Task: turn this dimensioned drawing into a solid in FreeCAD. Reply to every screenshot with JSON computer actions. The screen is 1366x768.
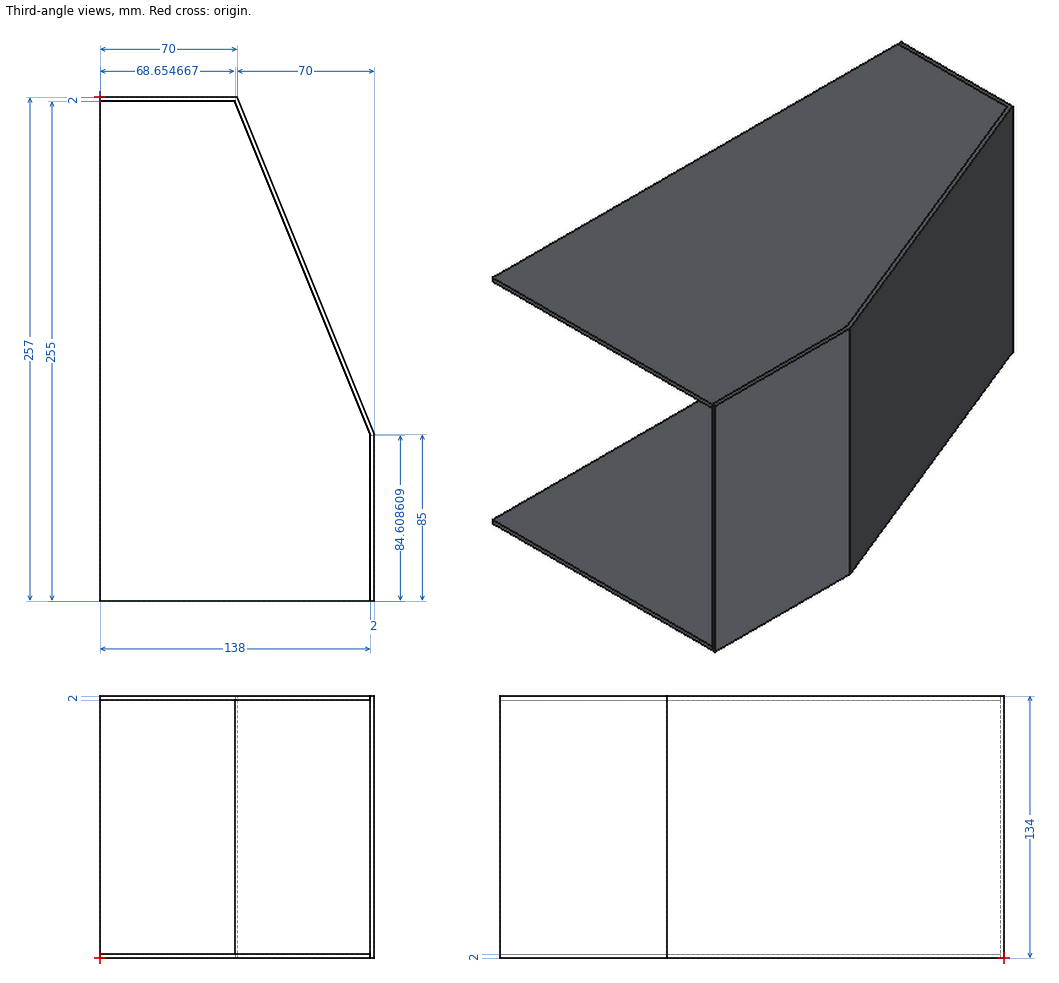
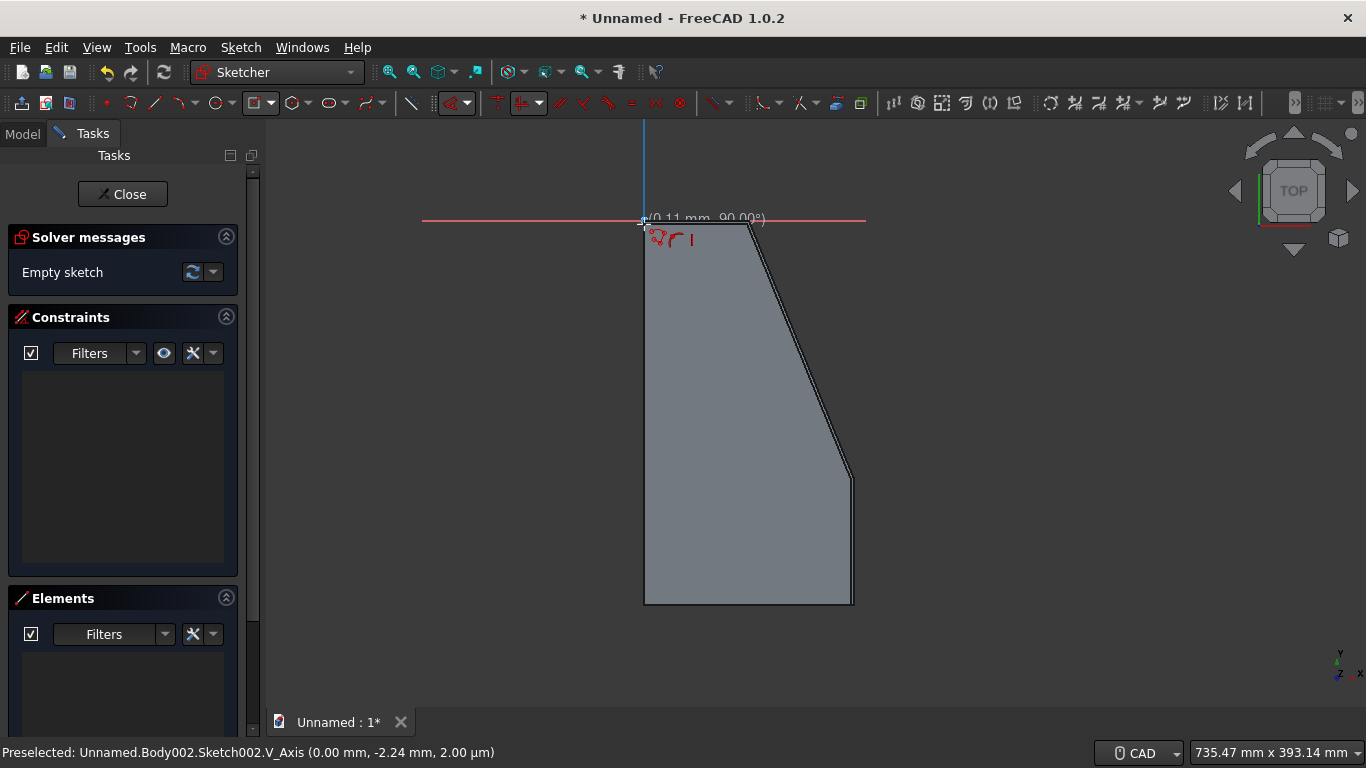
{"action": "left_click", "coordinate": [653, 605]}
{"action": "left_click", "coordinate": [851, 605]}
{"action": "left_click", "coordinate": [851, 479]}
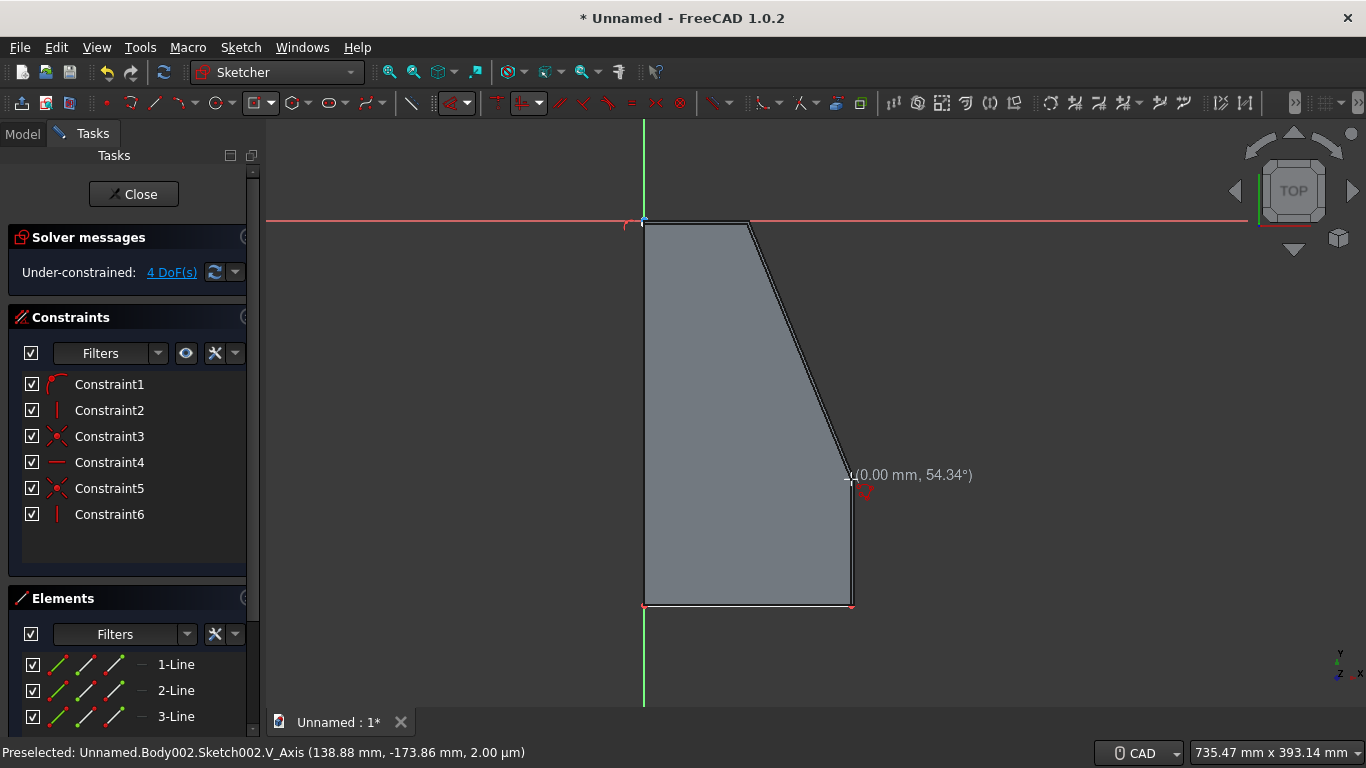
{"action": "scroll", "coordinate": [747, 224], "scroll_direction": "up", "scroll_amount": 9}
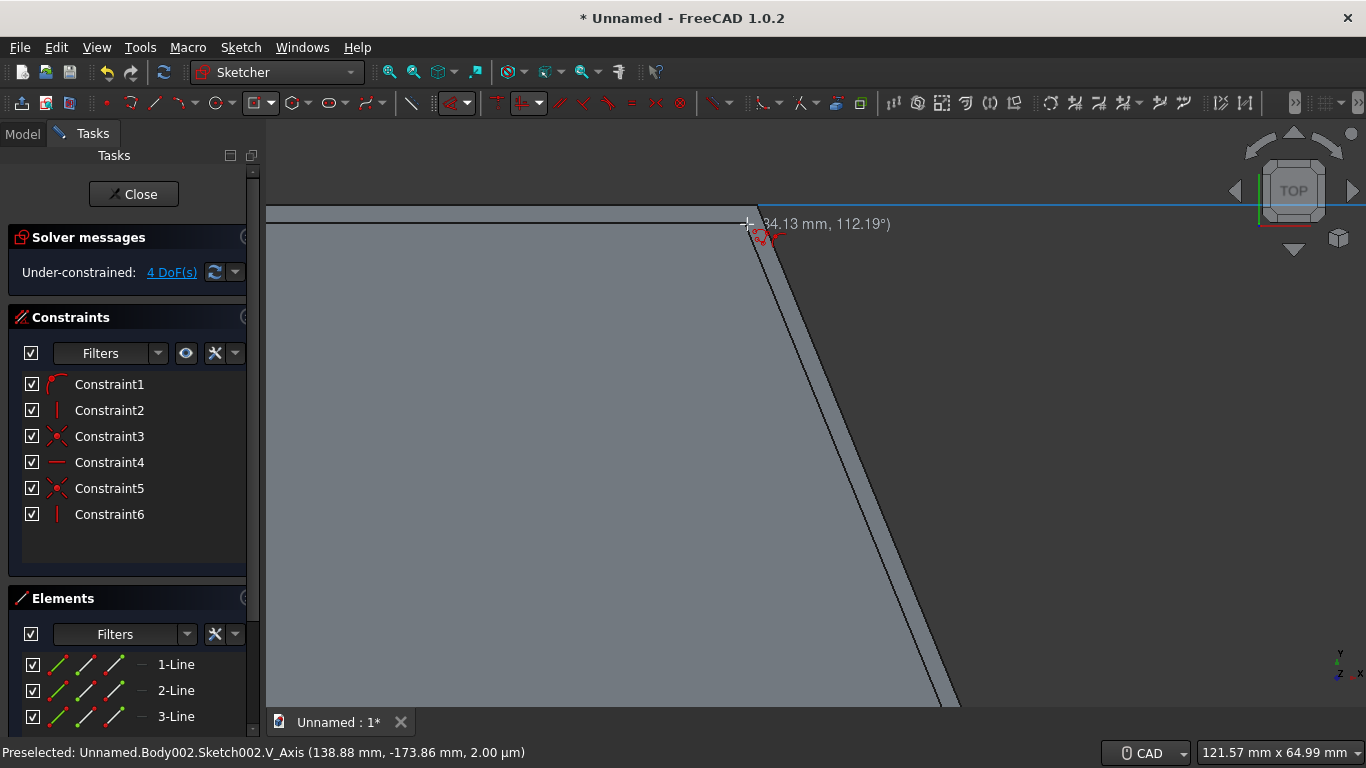
{"action": "left_click", "coordinate": [745, 223]}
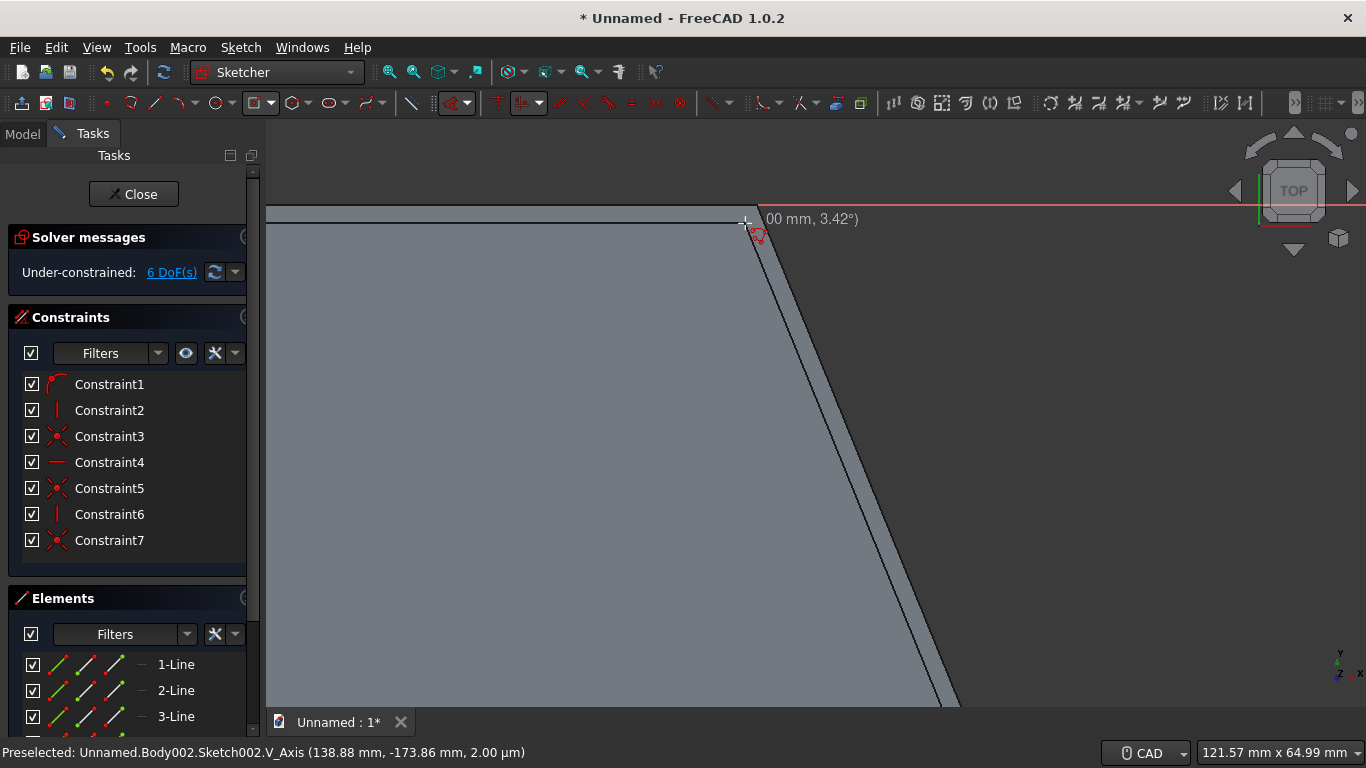
{"action": "scroll", "coordinate": [747, 224], "scroll_direction": "down", "scroll_amount": 9}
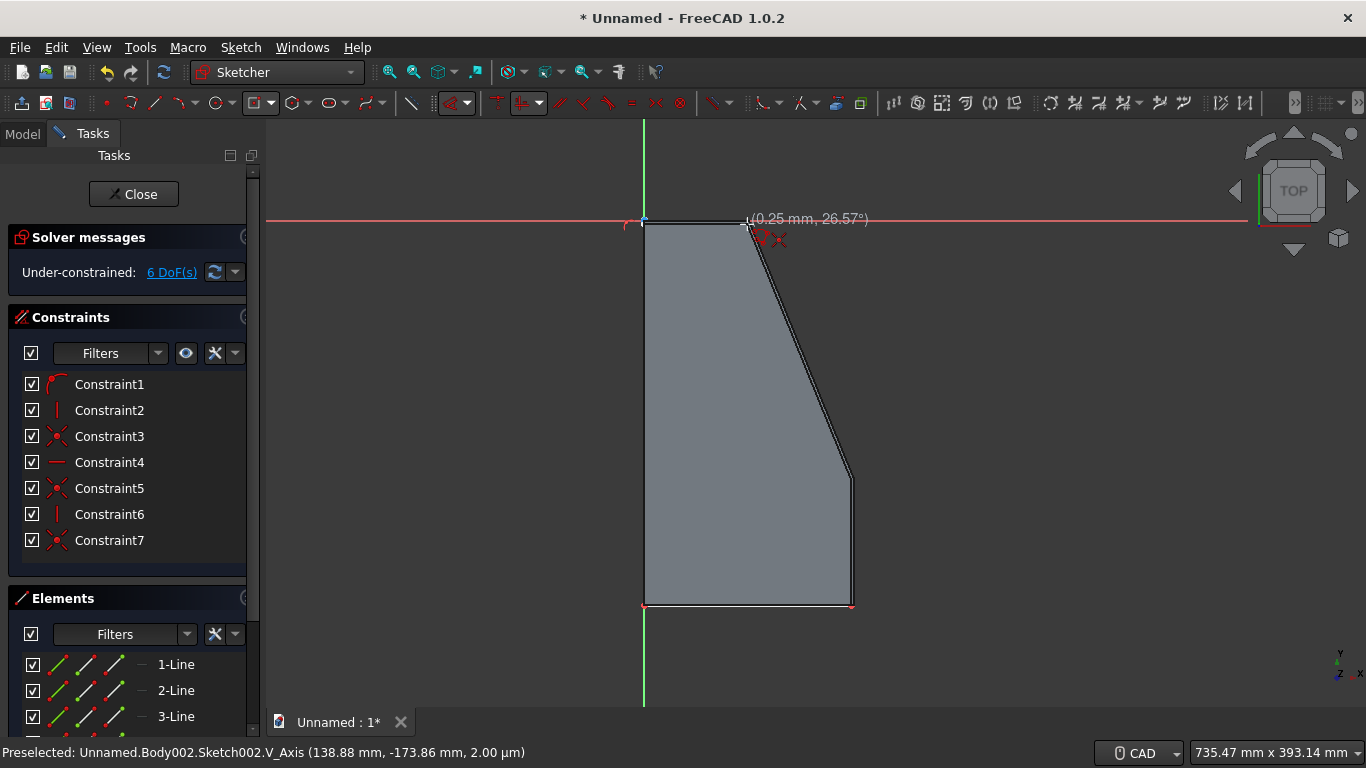
{"action": "scroll", "coordinate": [644, 224], "scroll_direction": "up", "scroll_amount": 9}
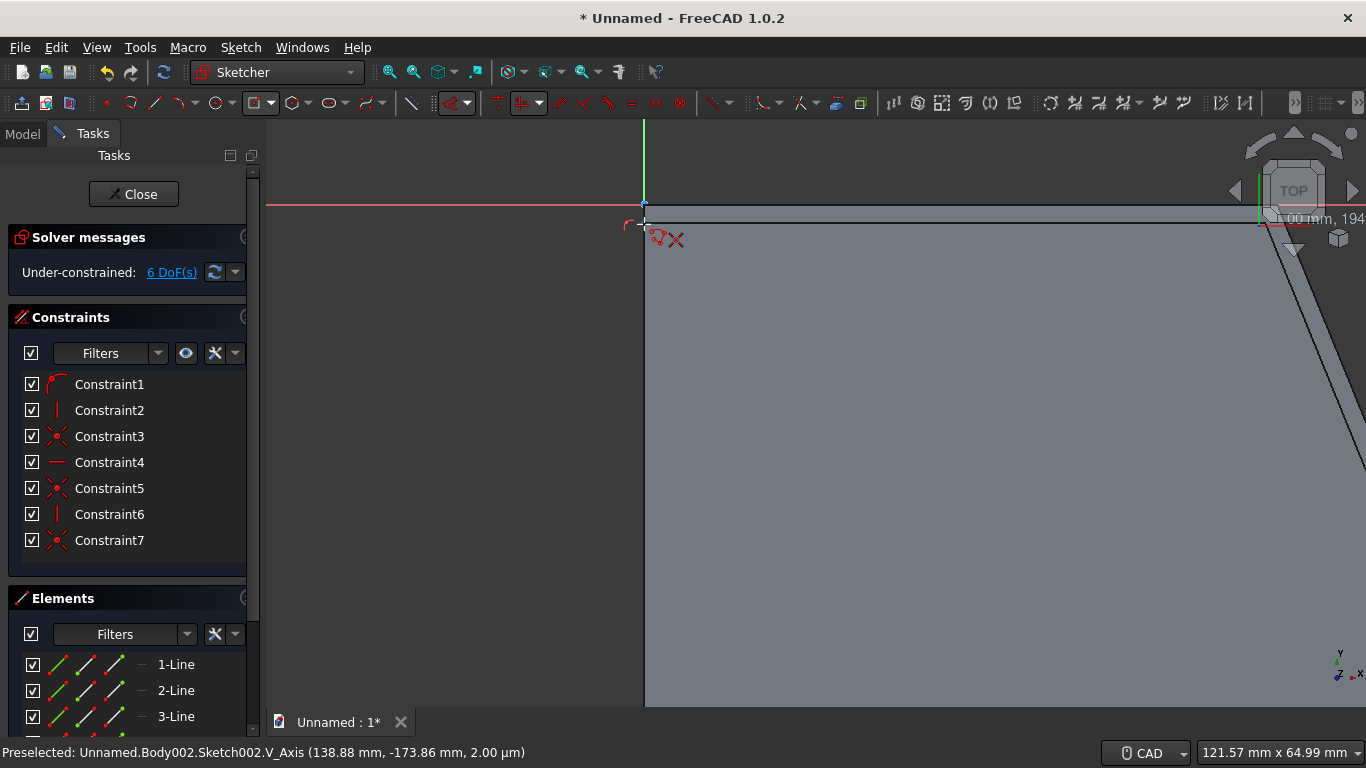
{"action": "left_click", "coordinate": [644, 224]}
{"action": "key", "text": "Escape"}
{"action": "key", "text": "Escape"}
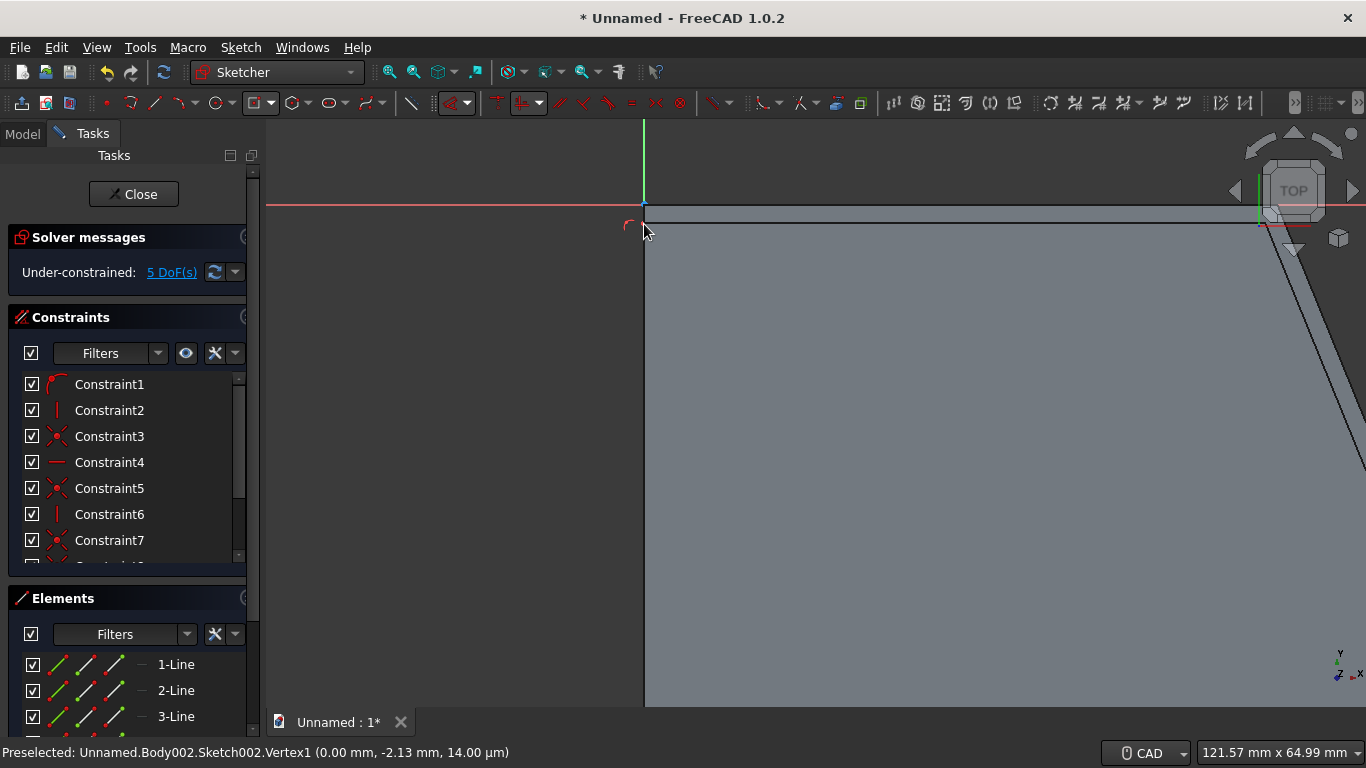
{"action": "key", "text": "d"}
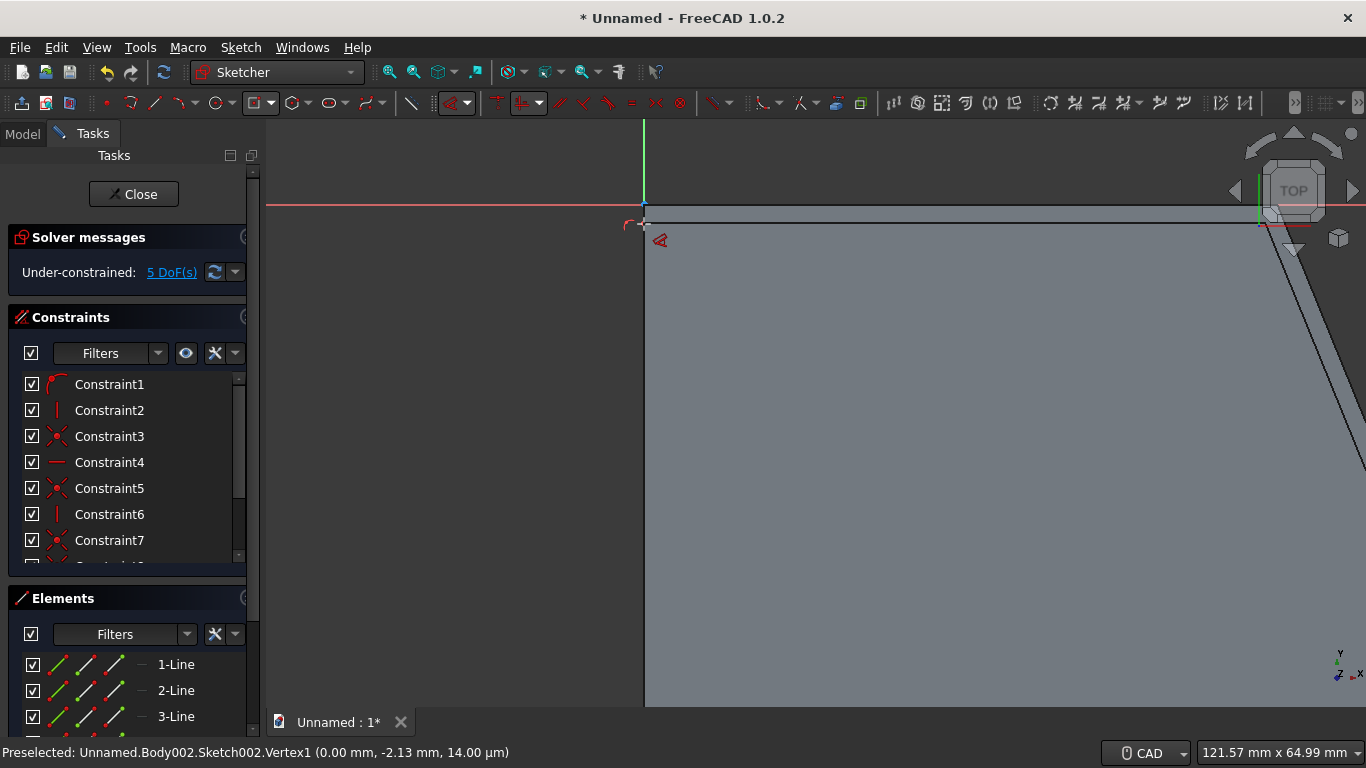
{"action": "scroll", "coordinate": [644, 224], "scroll_direction": "up", "scroll_amount": 4}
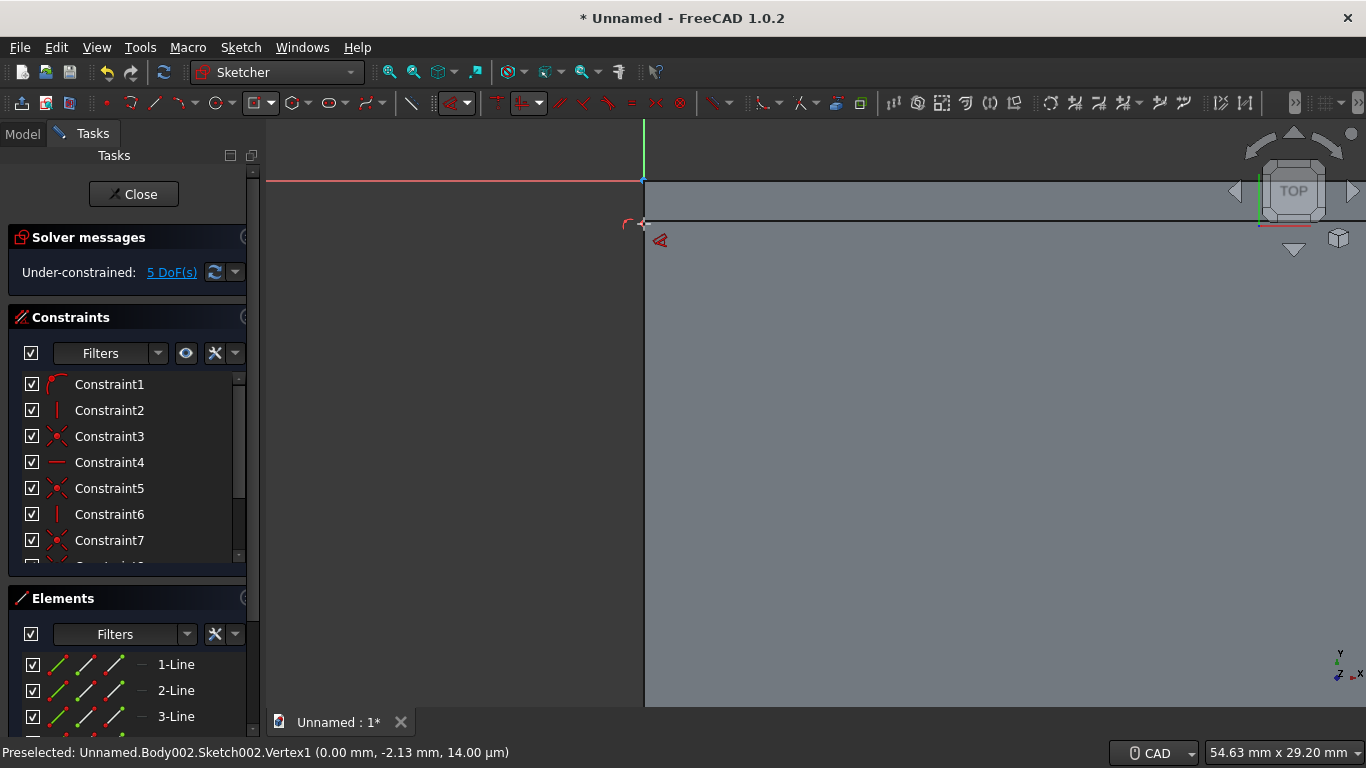
{"action": "left_click", "coordinate": [644, 224]}
{"action": "left_click", "coordinate": [610, 202]}